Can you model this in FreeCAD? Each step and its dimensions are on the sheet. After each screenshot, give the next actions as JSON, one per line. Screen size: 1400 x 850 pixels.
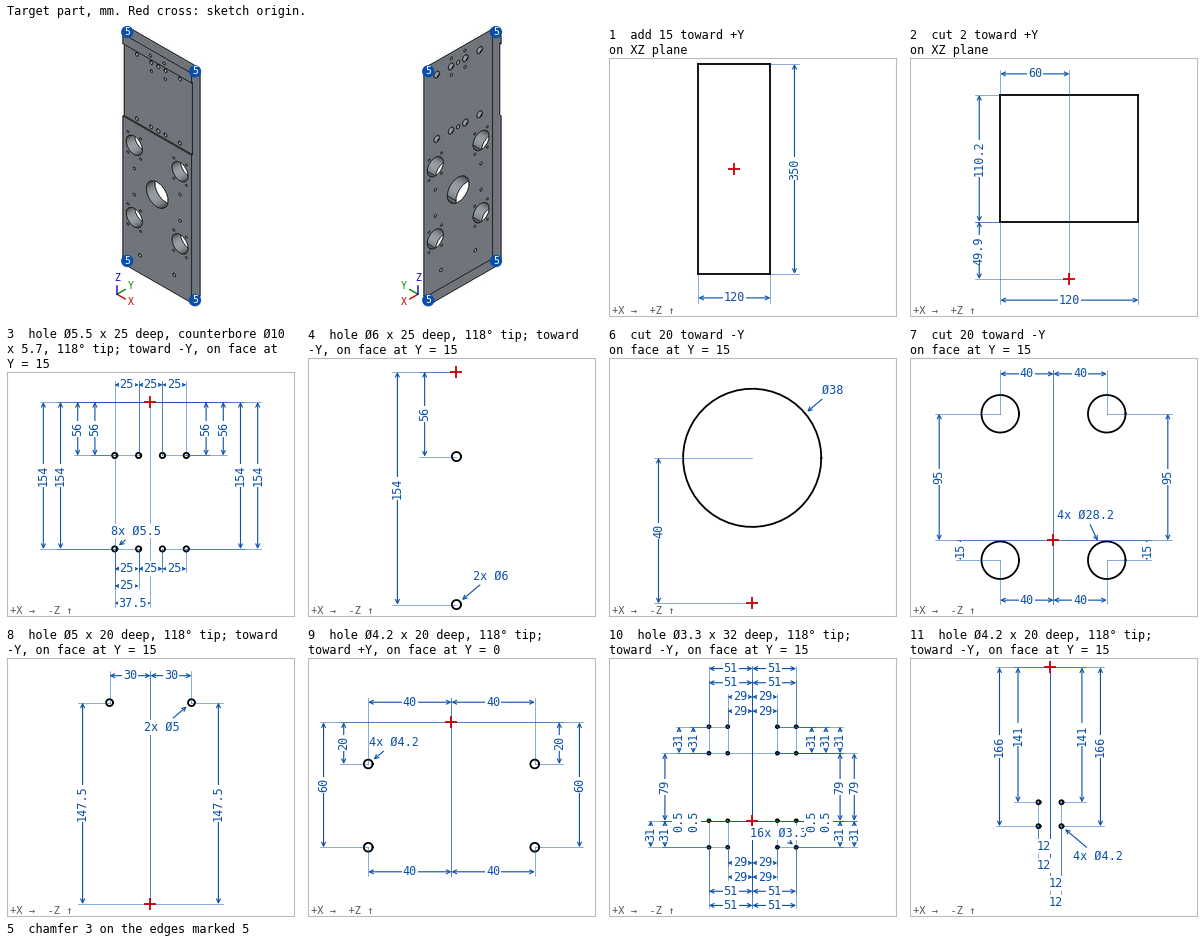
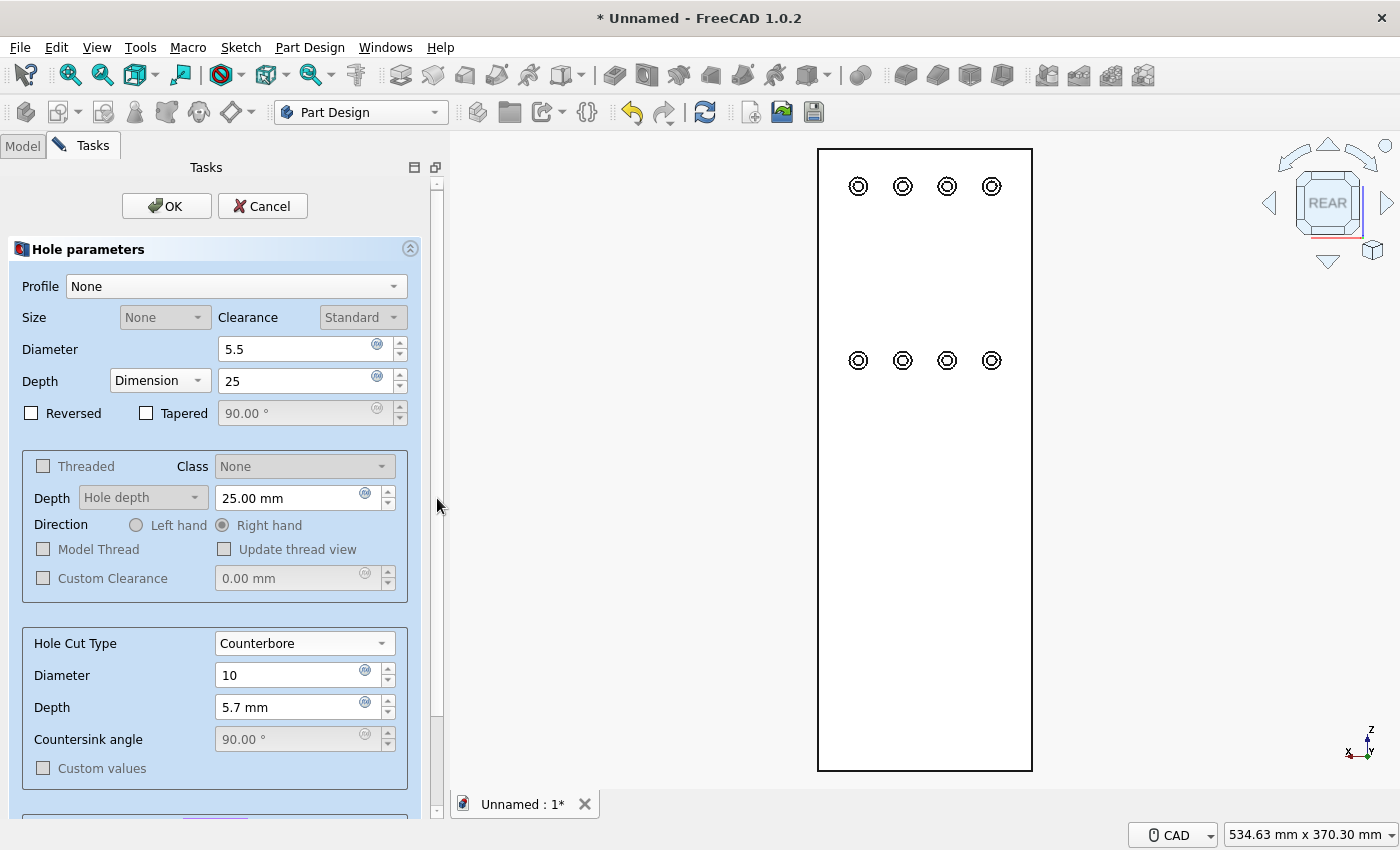
{"action": "left_click", "coordinate": [167, 206]}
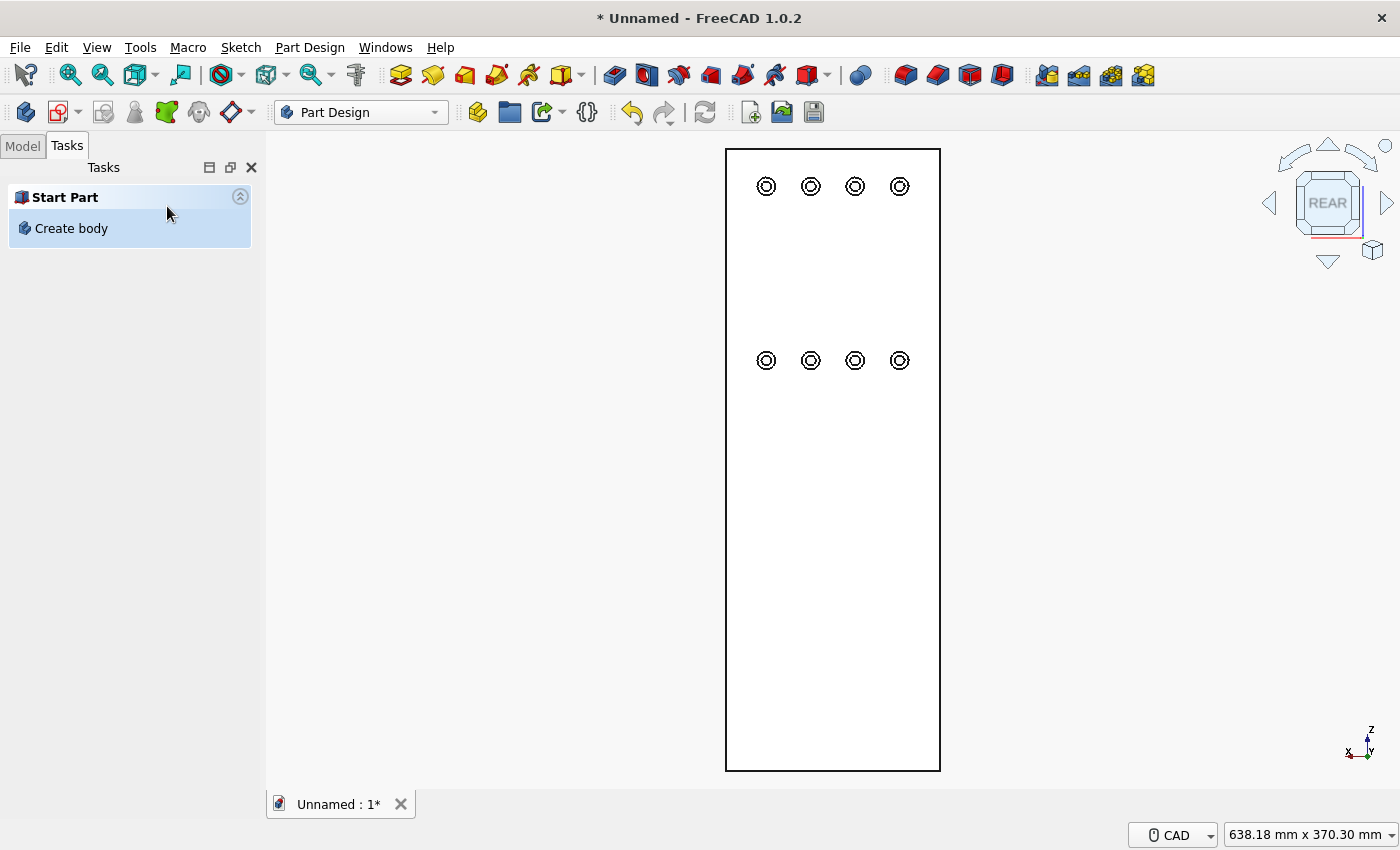
{"action": "left_click", "coordinate": [833, 548]}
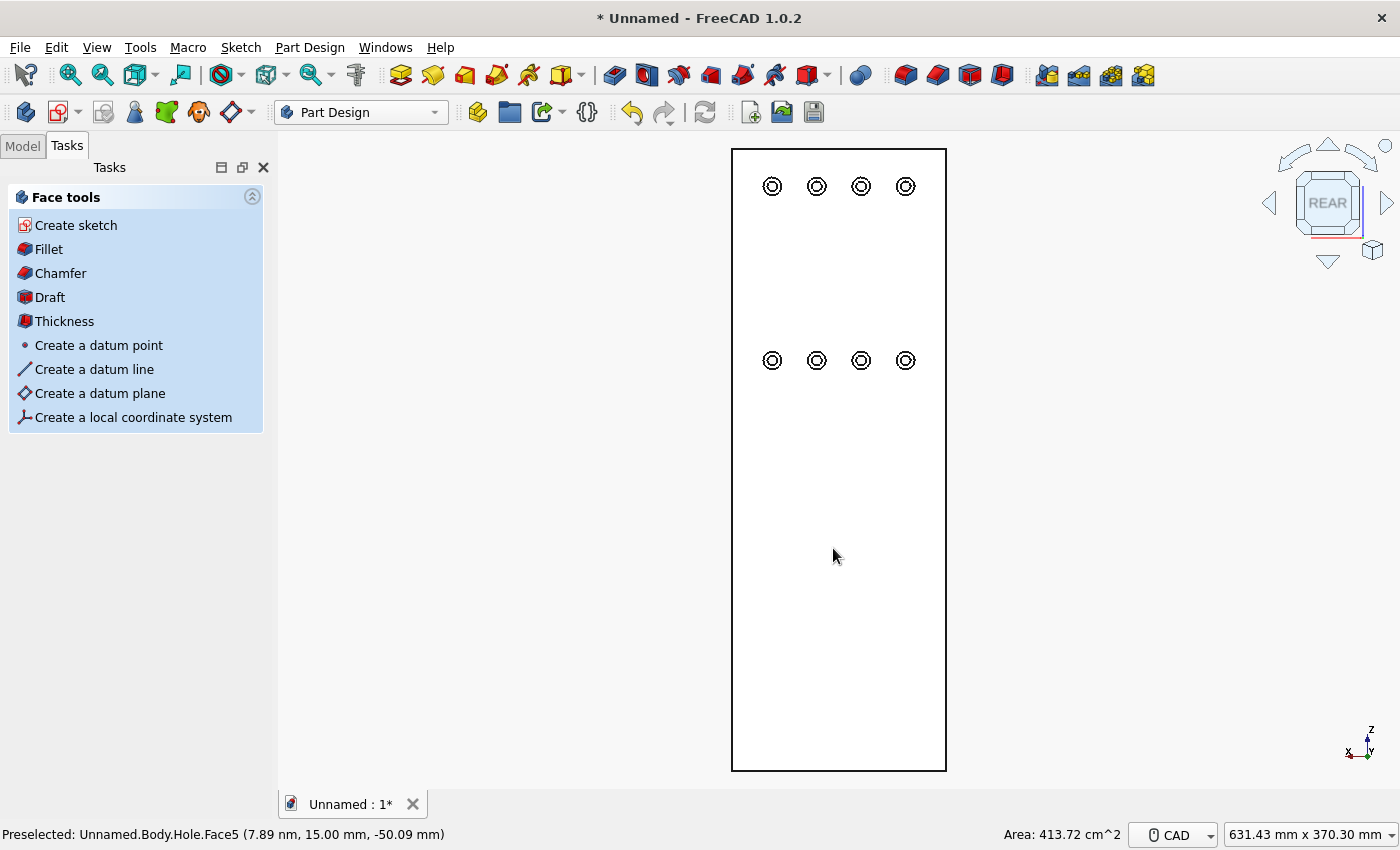
{"action": "left_click", "coordinate": [58, 112]}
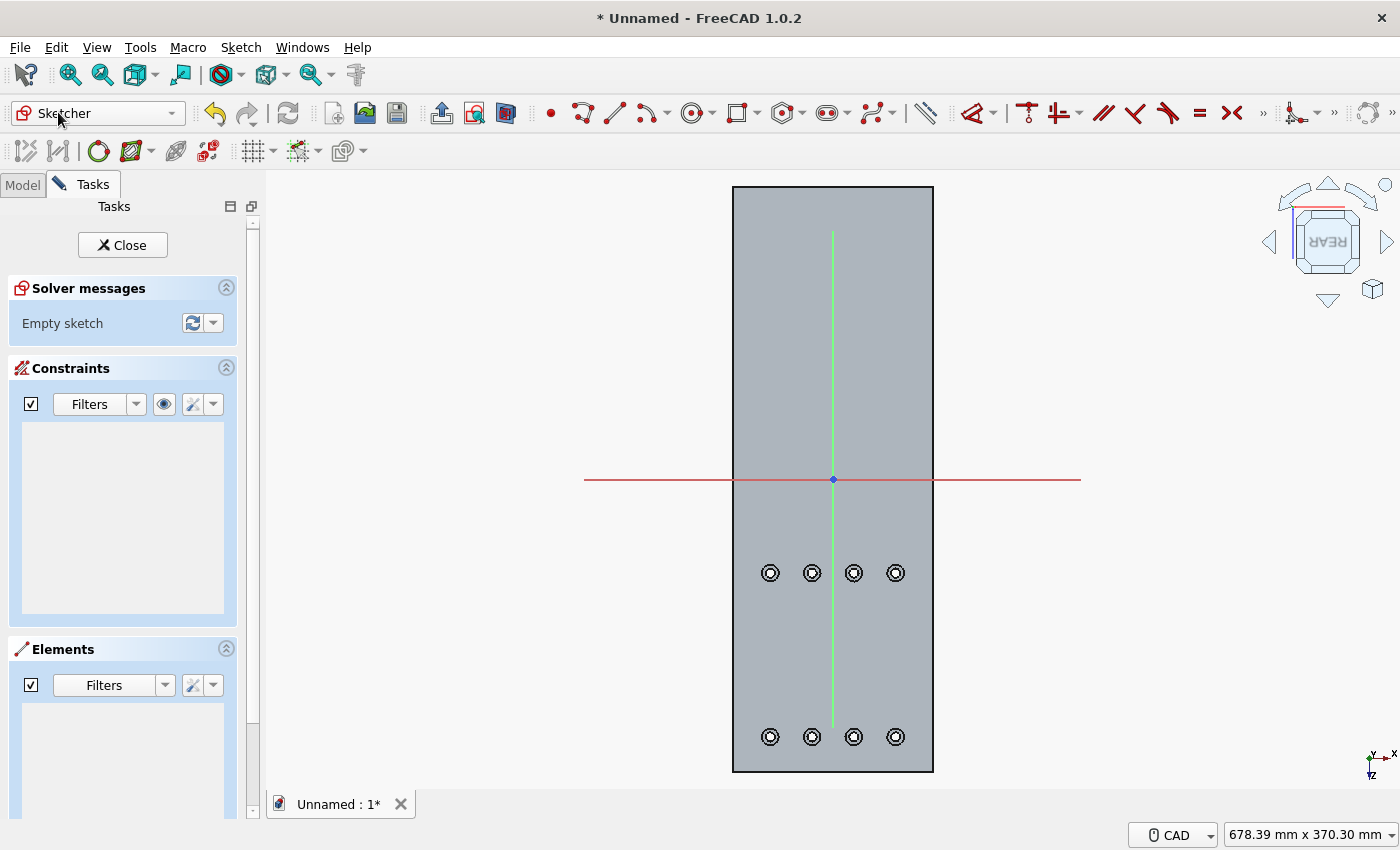
{"action": "scroll", "coordinate": [972, 761], "scroll_direction": "up", "scroll_amount": 2}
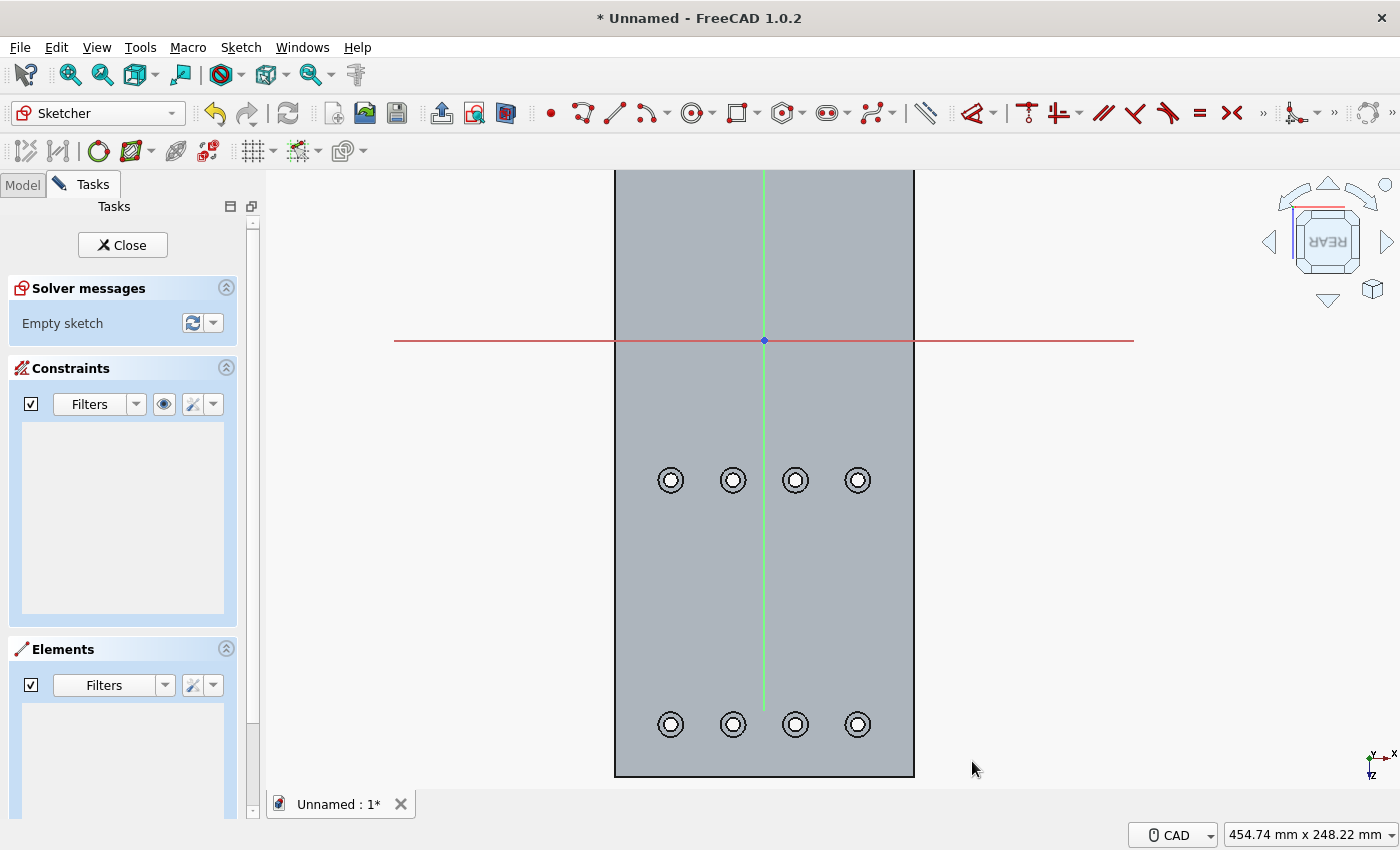
{"action": "left_click", "coordinate": [692, 114]}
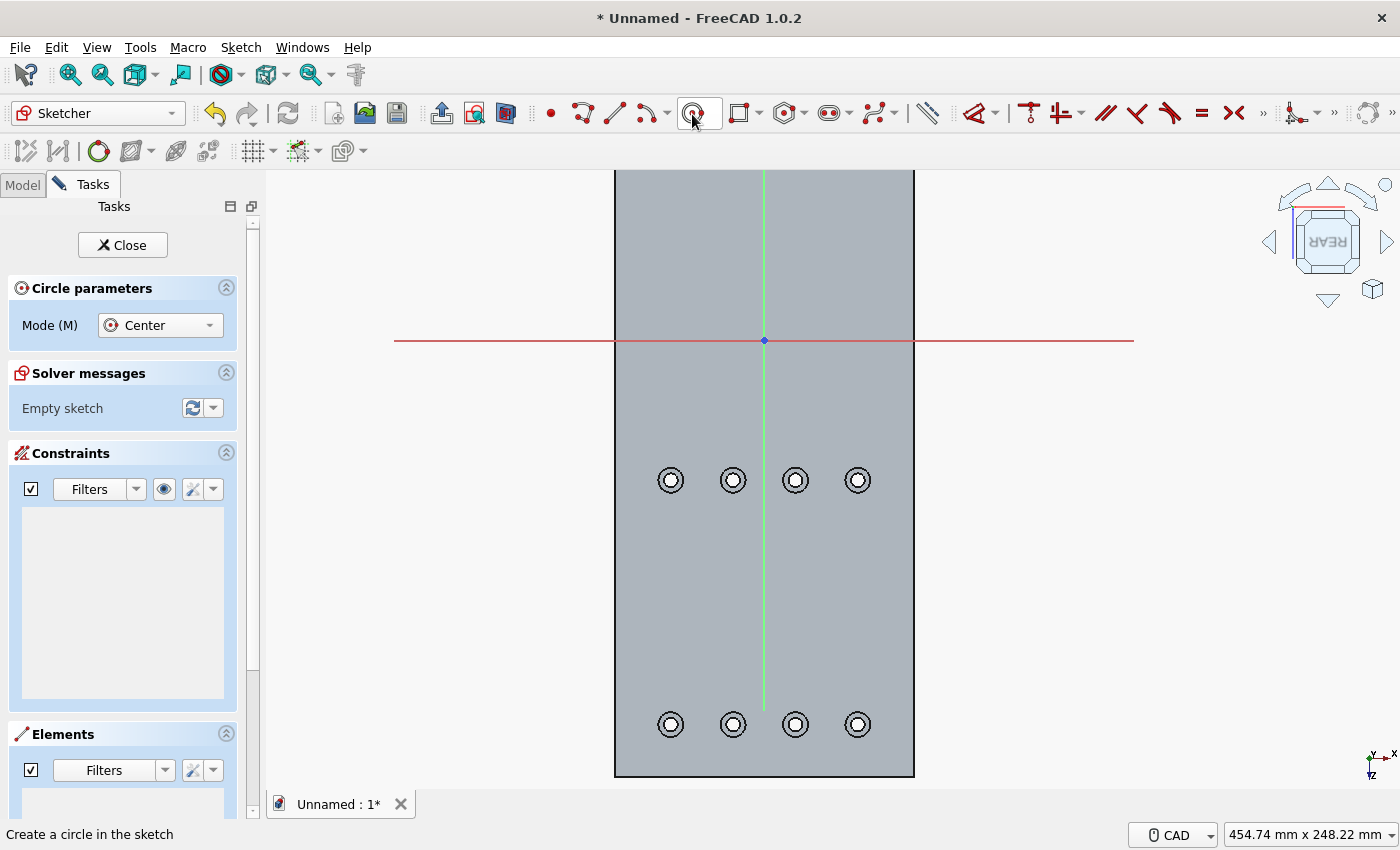
{"action": "scroll", "coordinate": [764, 725], "scroll_direction": "up", "scroll_amount": 6}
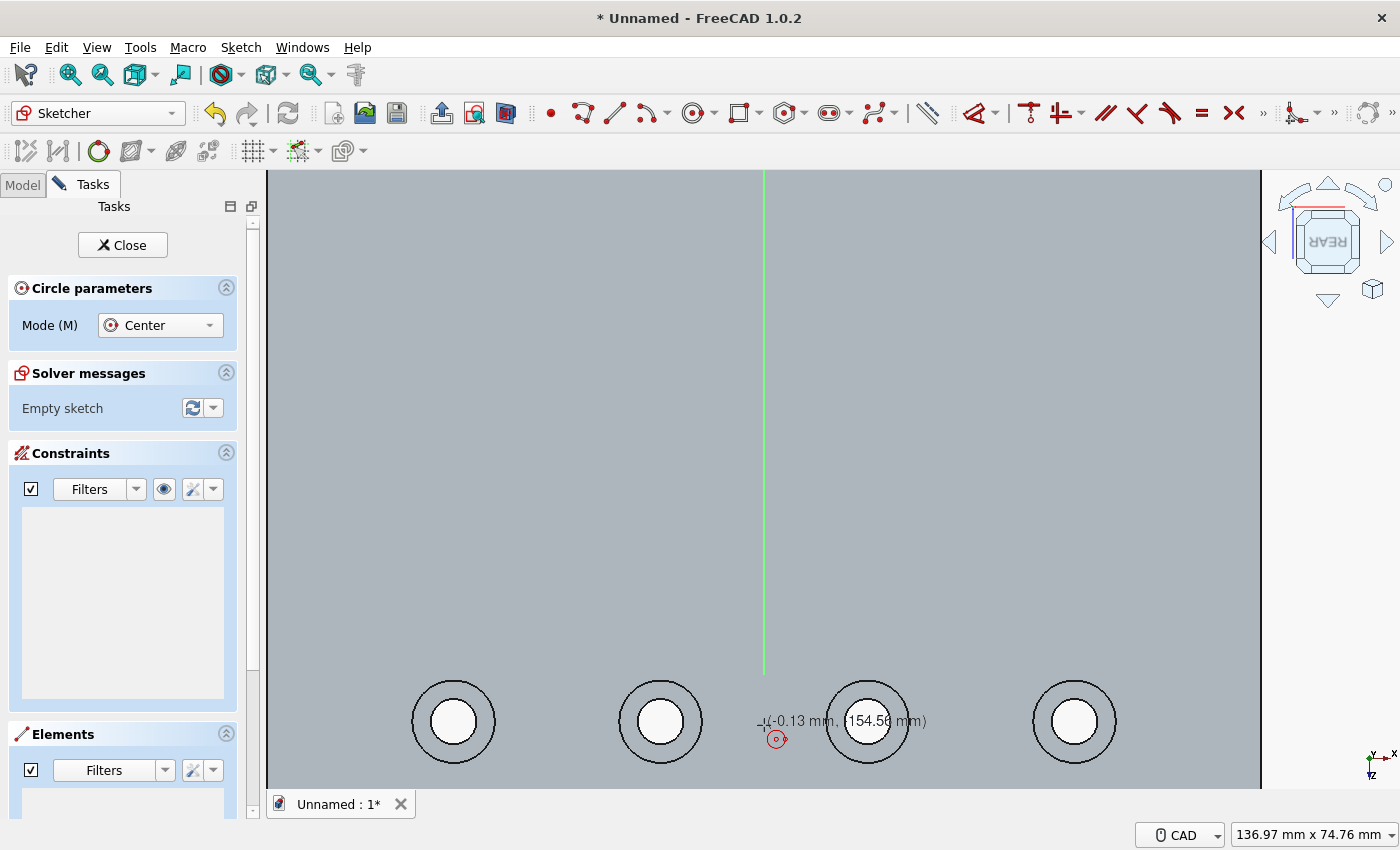
{"action": "left_click", "coordinate": [764, 722]}
{"action": "left_click", "coordinate": [782, 704]}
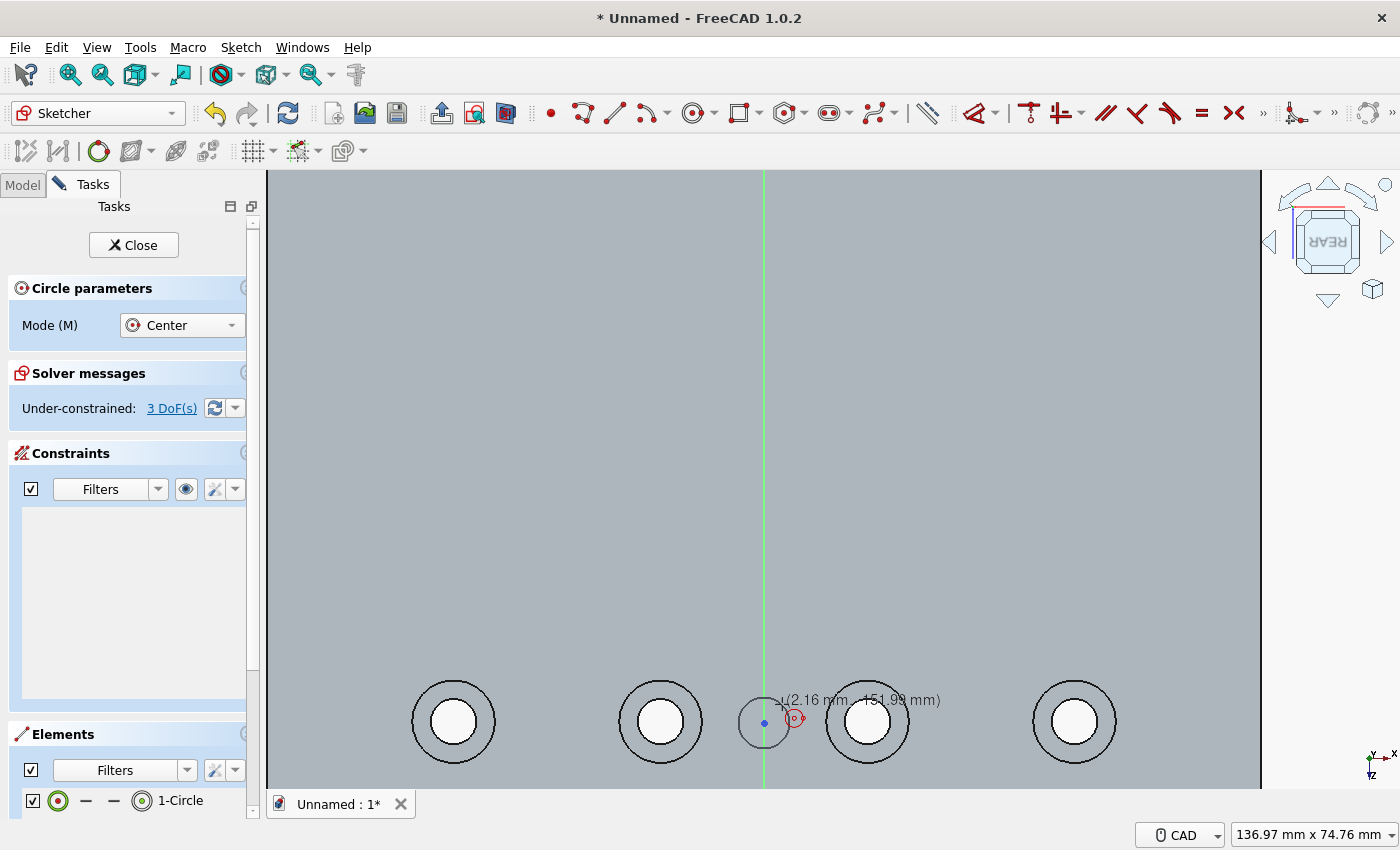
{"action": "scroll", "coordinate": [765, 645], "scroll_direction": "down", "scroll_amount": 6}